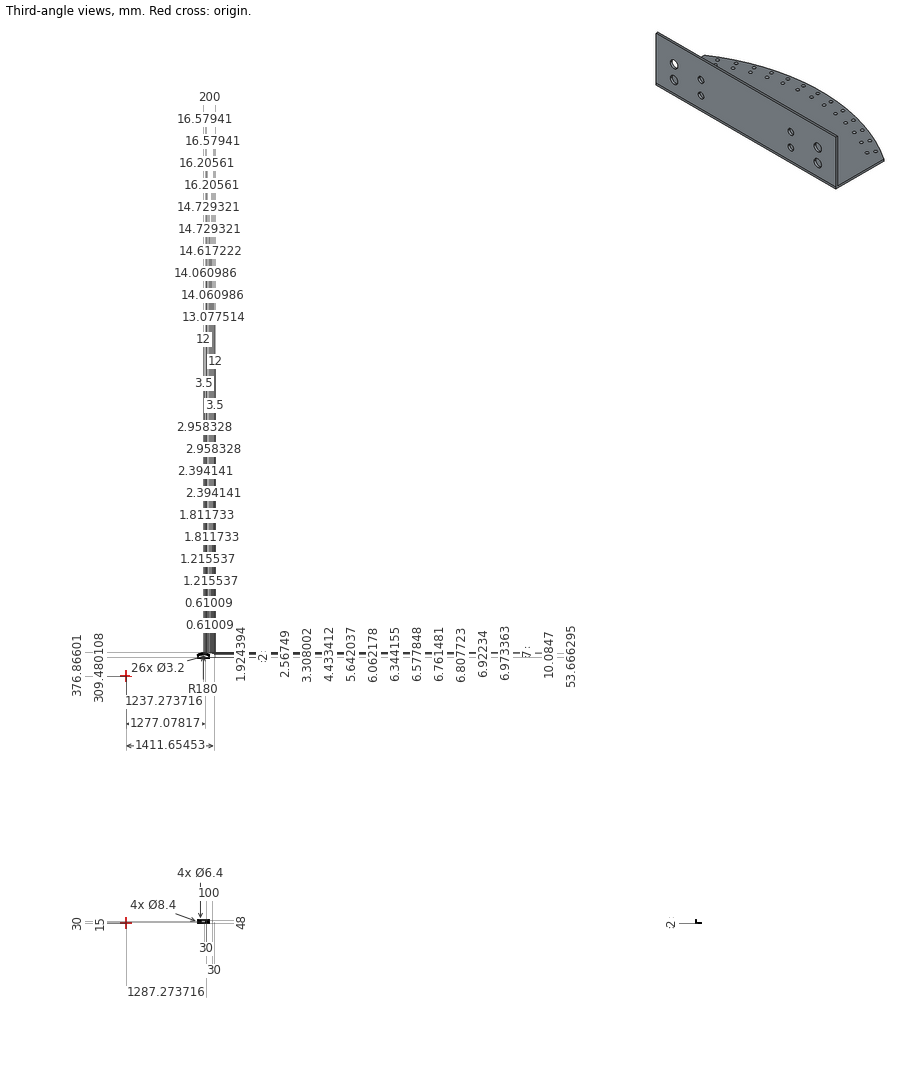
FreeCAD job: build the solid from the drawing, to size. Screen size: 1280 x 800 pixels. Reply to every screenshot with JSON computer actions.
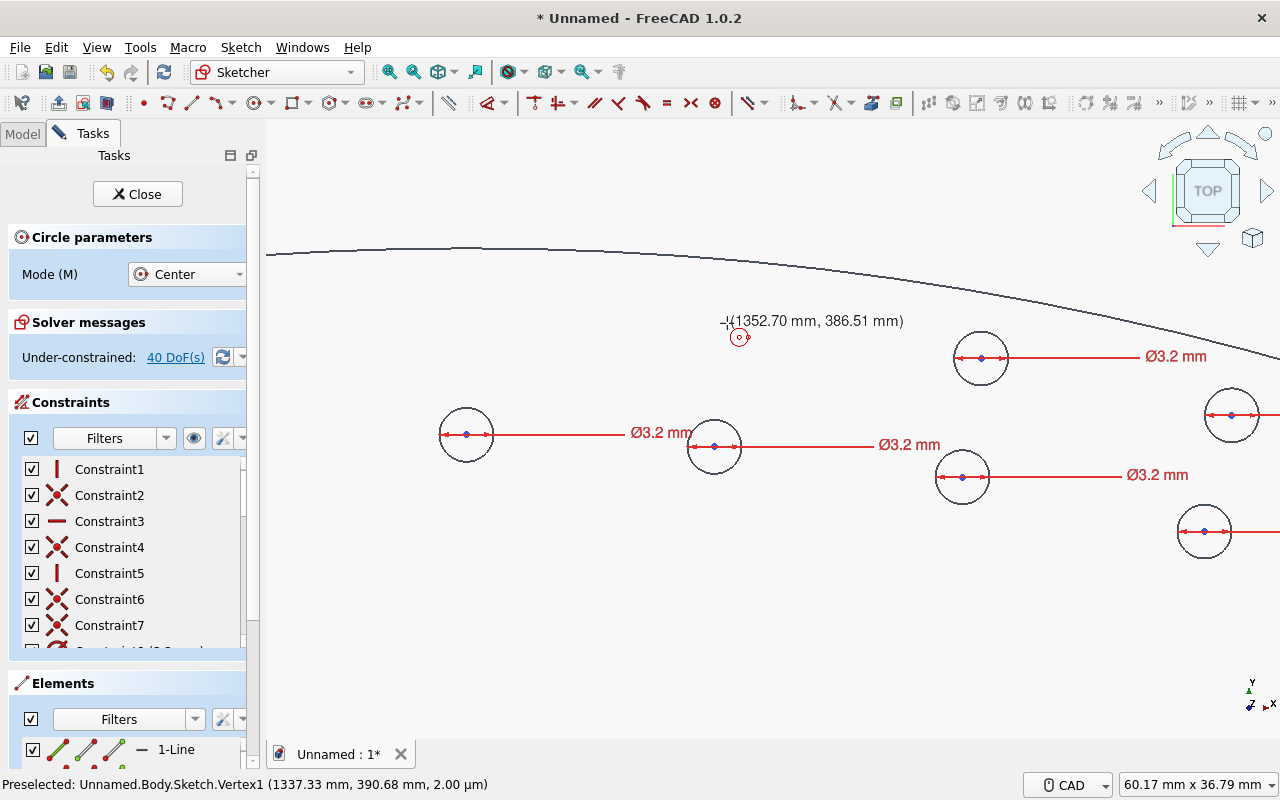
{"action": "scroll", "coordinate": [752, 326], "scroll_direction": "down", "scroll_amount": 9}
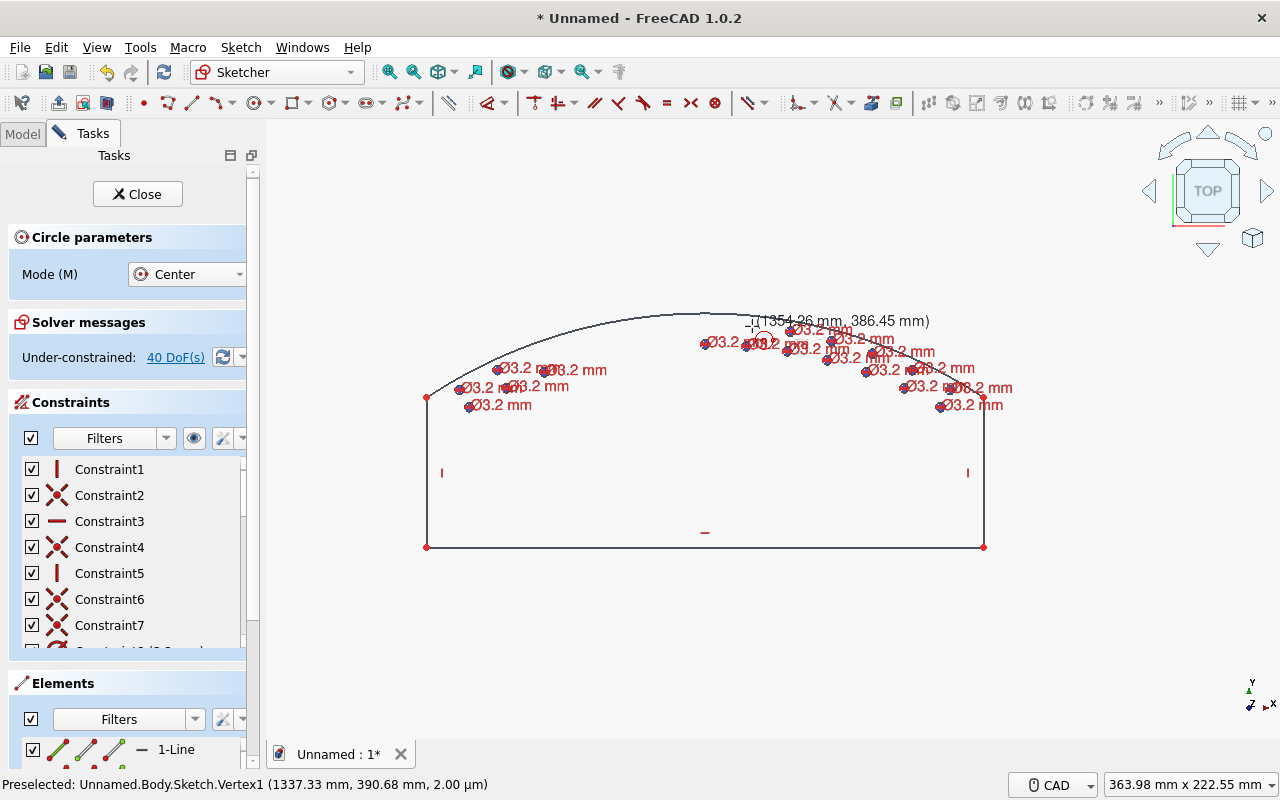
{"action": "scroll", "coordinate": [748, 325], "scroll_direction": "up", "scroll_amount": 2}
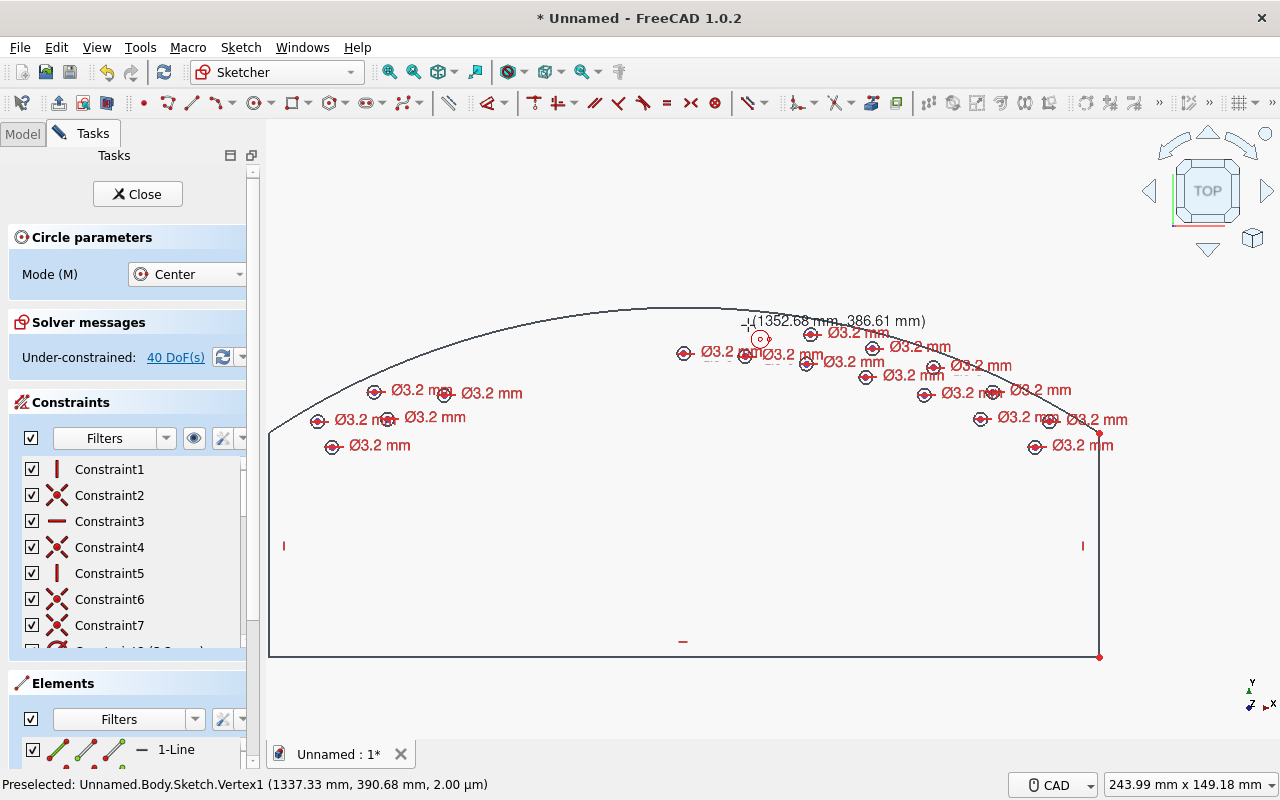
{"action": "left_click", "coordinate": [747, 326]}
{"action": "mouse_move", "coordinate": [752, 330]}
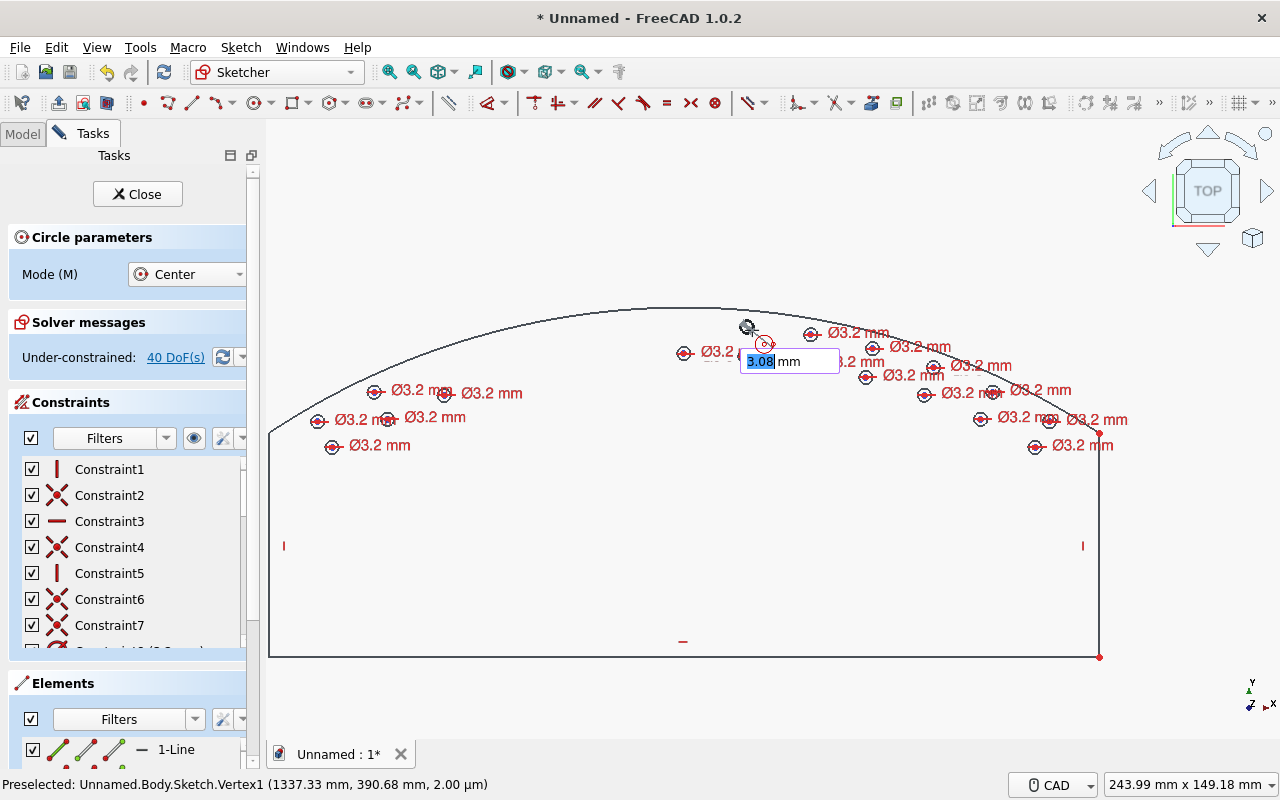
{"action": "type", "text": "3.2"}
{"action": "key", "text": "Return"}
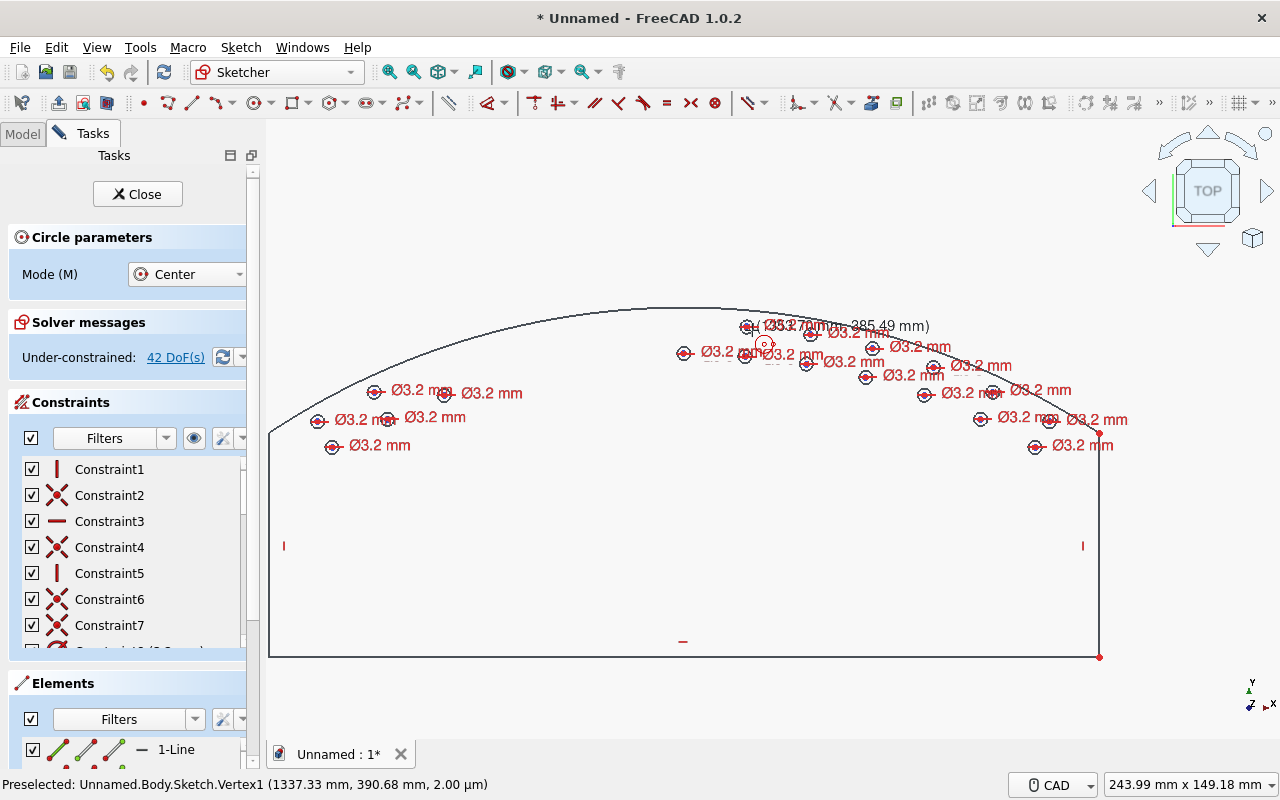
{"action": "scroll", "coordinate": [684, 323], "scroll_direction": "up", "scroll_amount": 7}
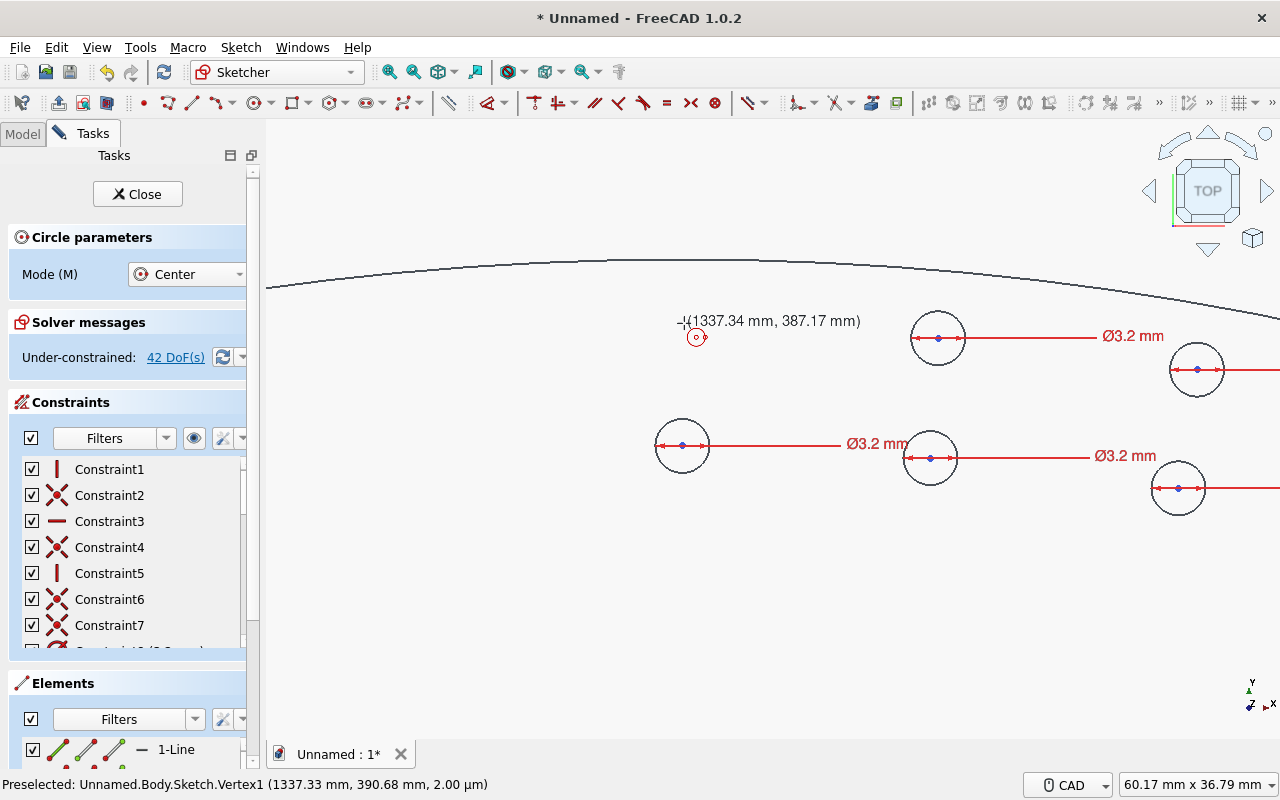
{"action": "scroll", "coordinate": [709, 324], "scroll_direction": "down", "scroll_amount": 9}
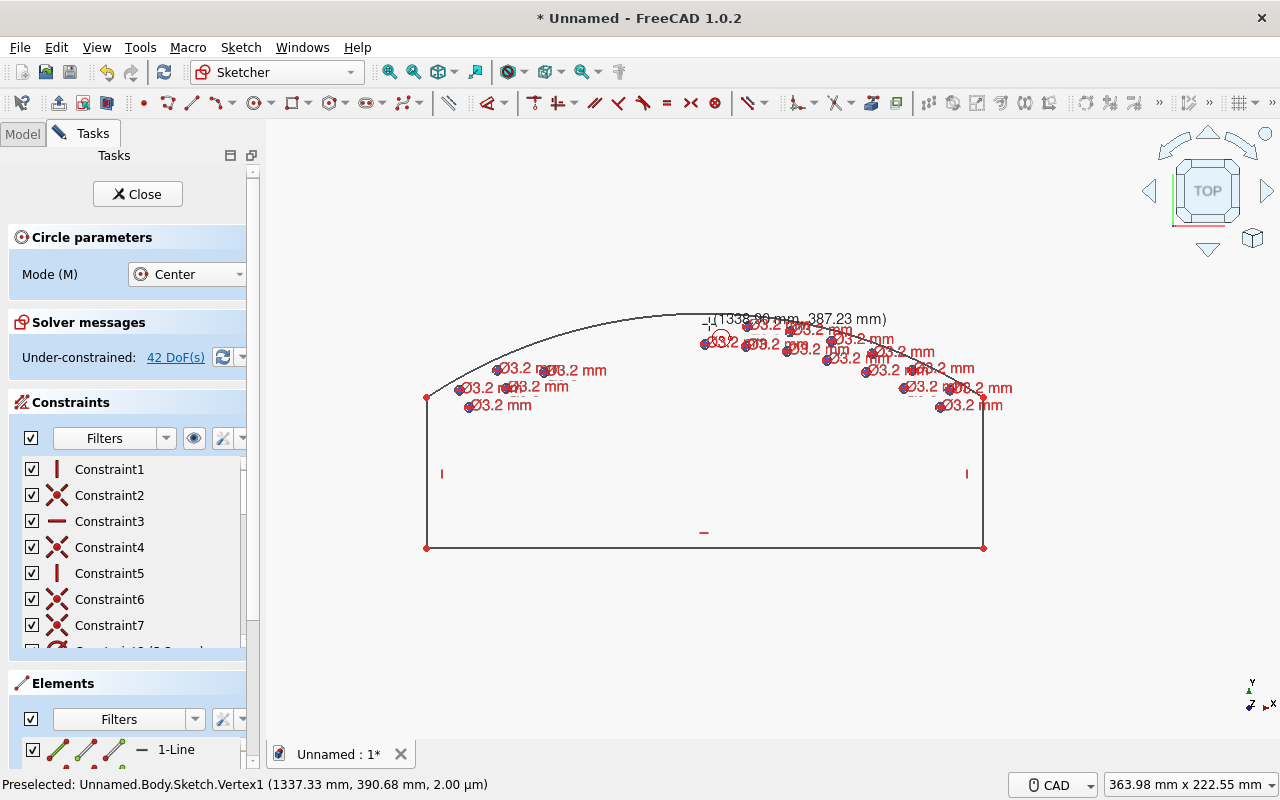
{"action": "scroll", "coordinate": [705, 324], "scroll_direction": "up", "scroll_amount": 2}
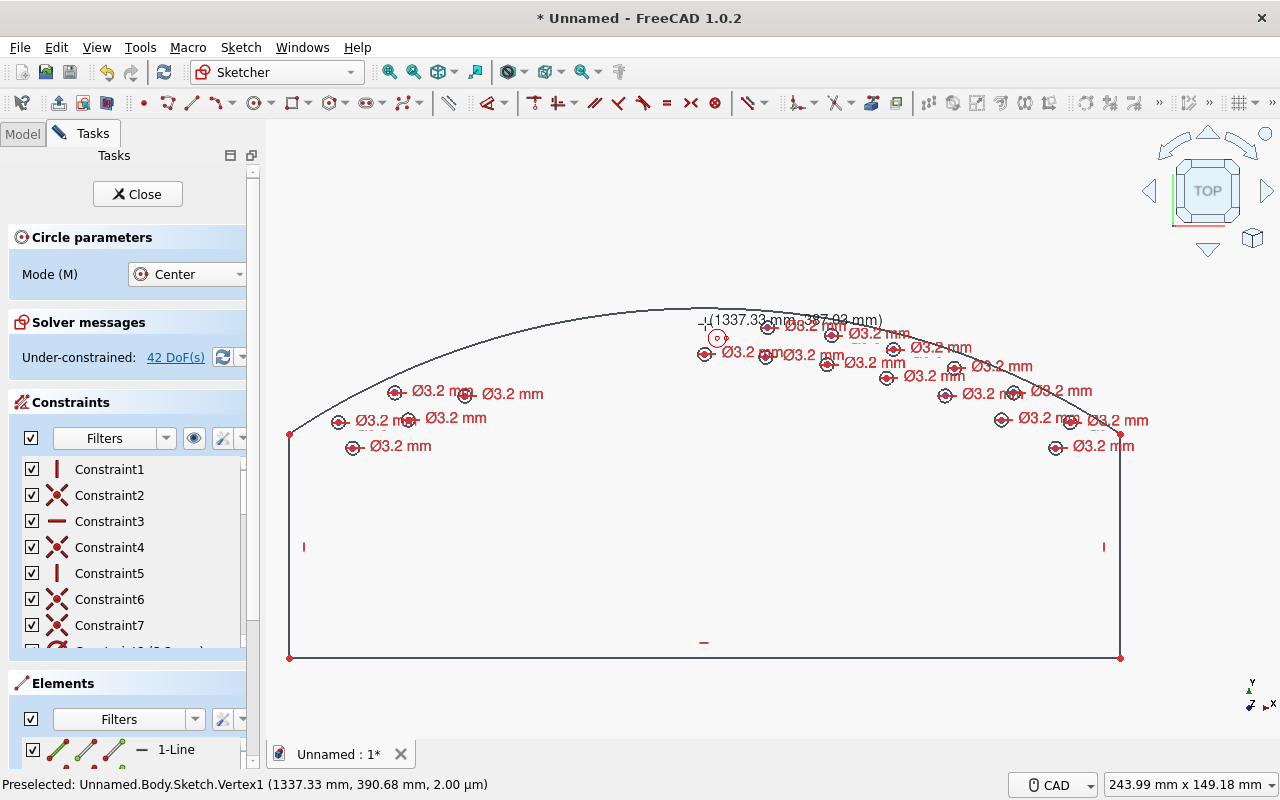
{"action": "left_click", "coordinate": [705, 323]}
{"action": "mouse_move", "coordinate": [709, 328]}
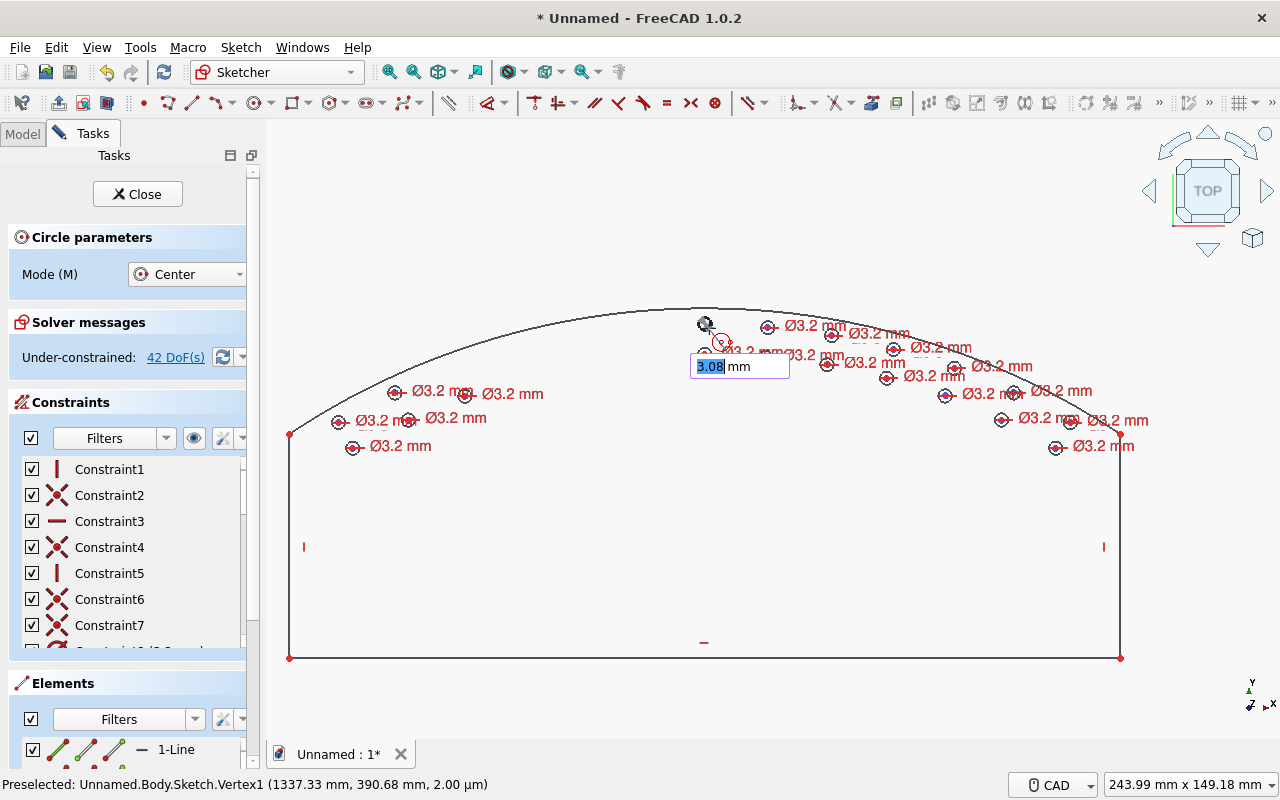
{"action": "type", "text": "3.2"}
{"action": "key", "text": "Return"}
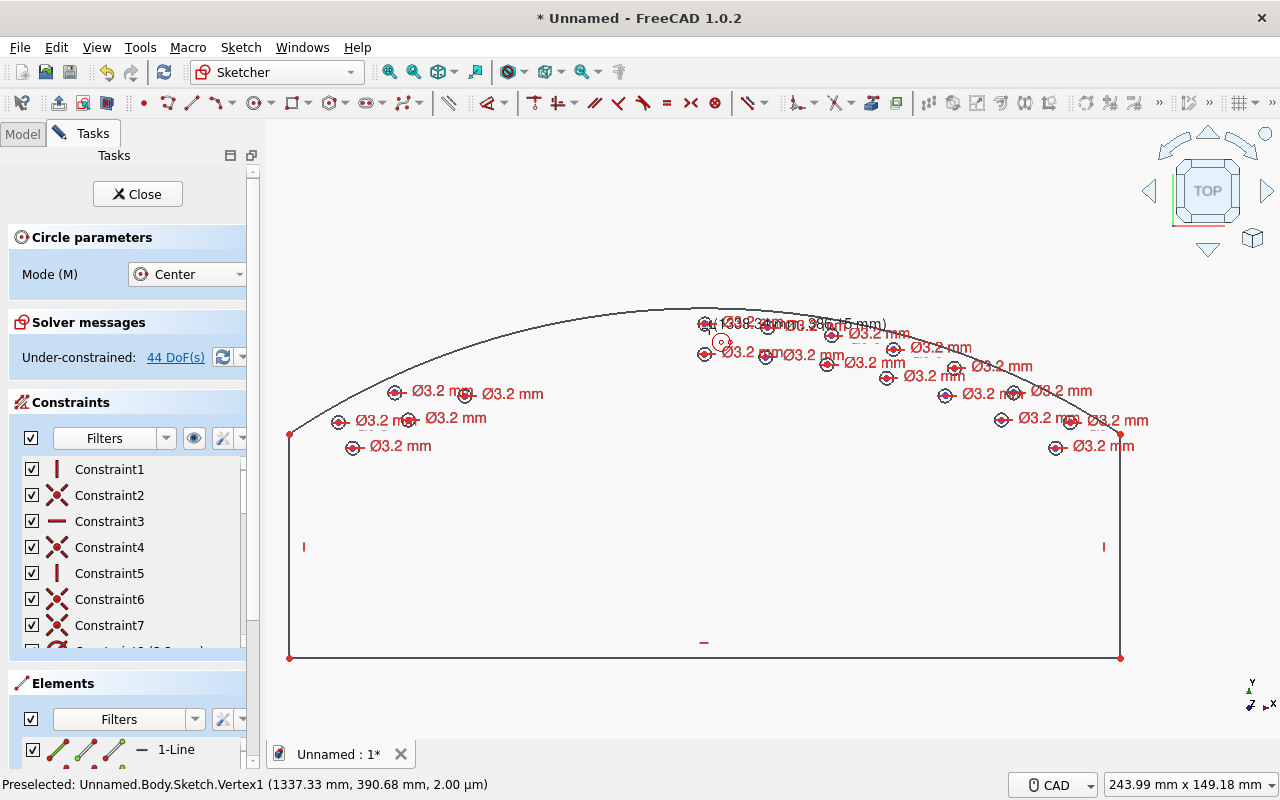
{"action": "scroll", "coordinate": [523, 376], "scroll_direction": "up", "scroll_amount": 7}